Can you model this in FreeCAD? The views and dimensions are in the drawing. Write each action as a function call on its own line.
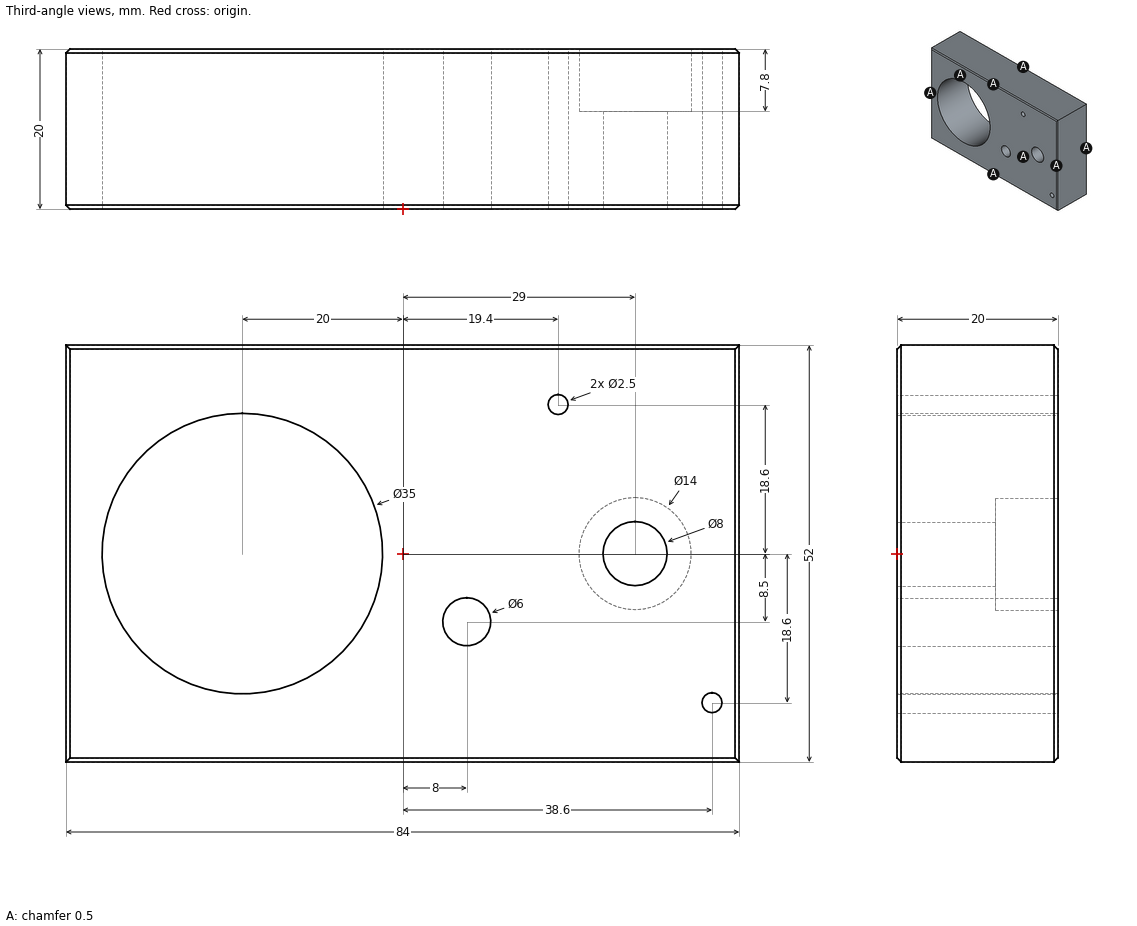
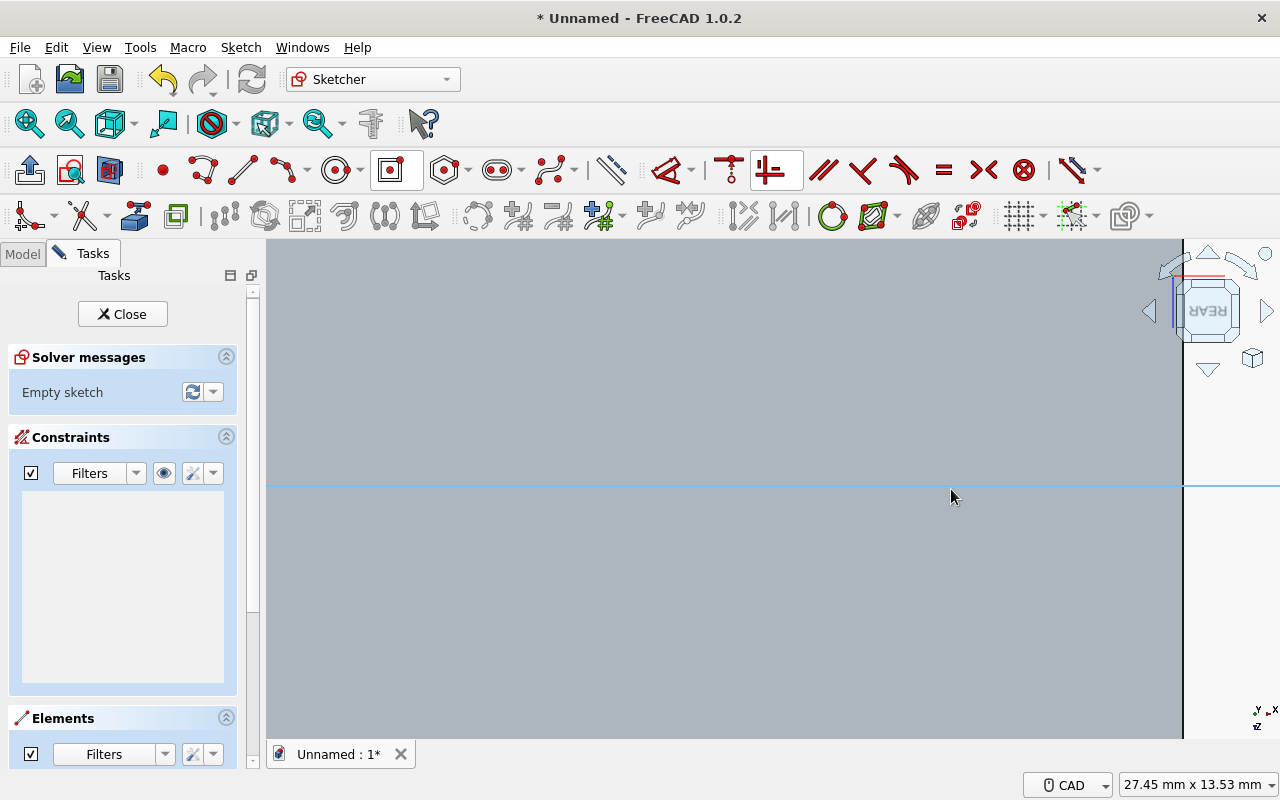
click(336, 170)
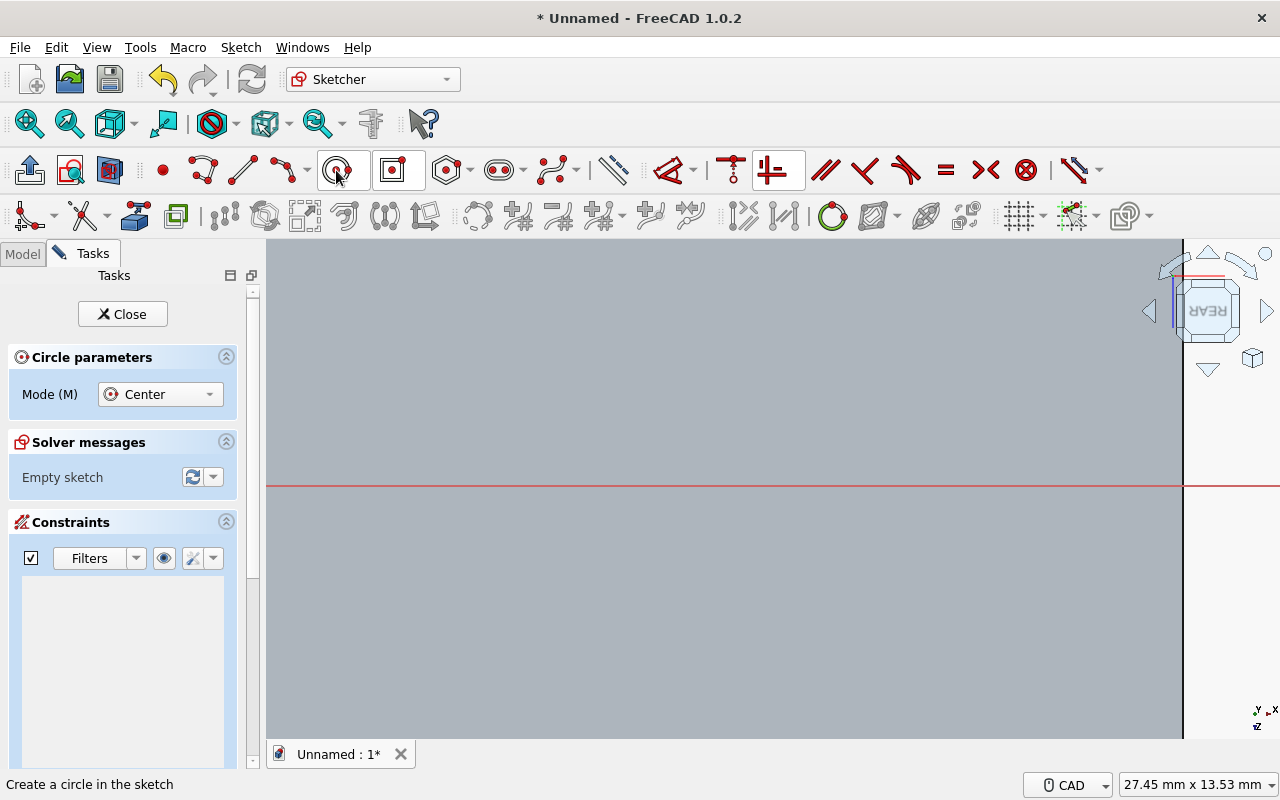
click(703, 486)
move(807, 381)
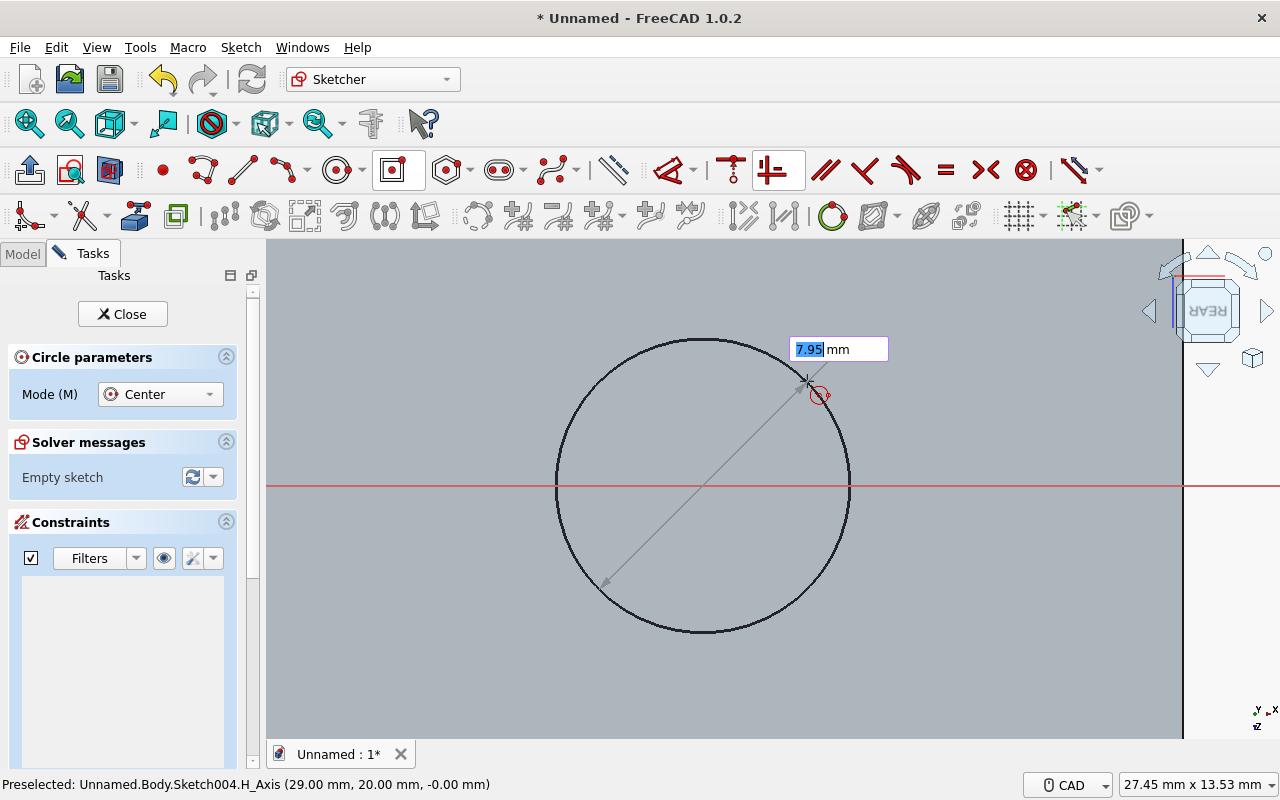
text(8)
key(Return)
key(Escape)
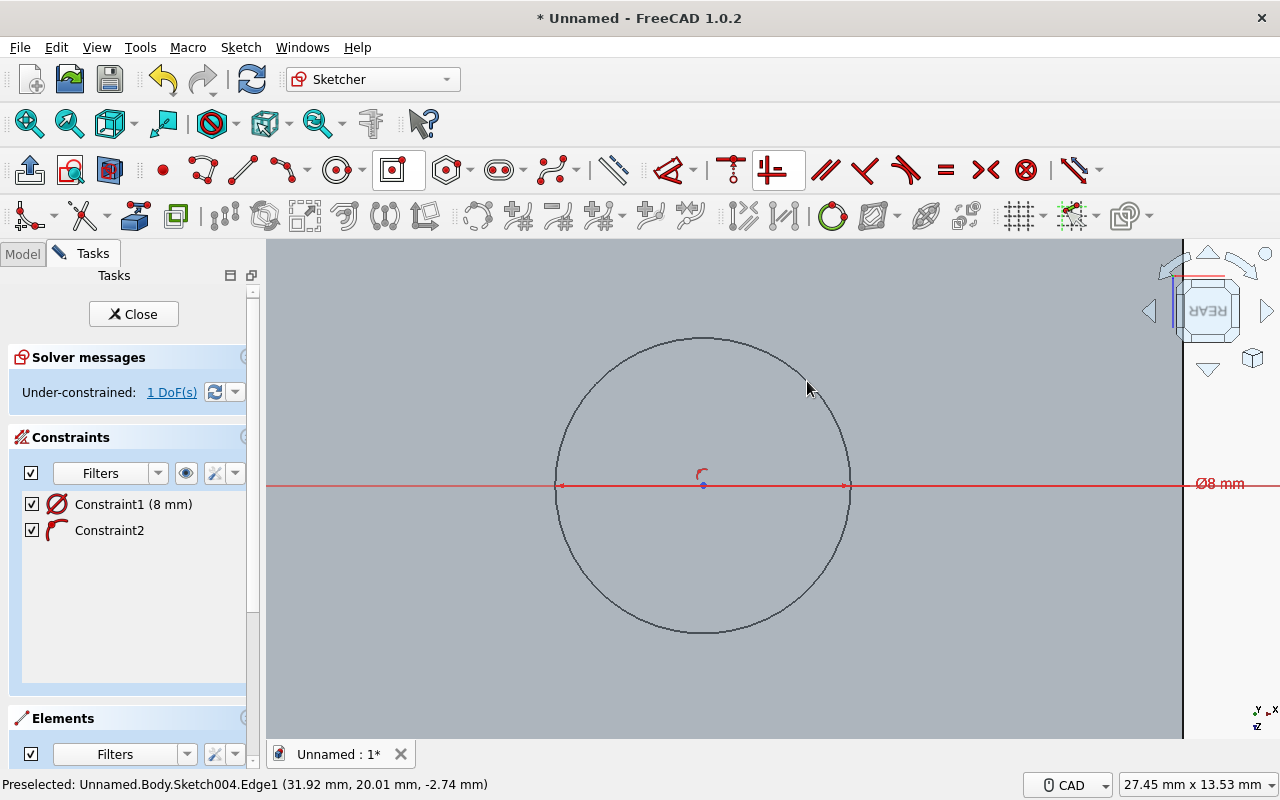
click(668, 170)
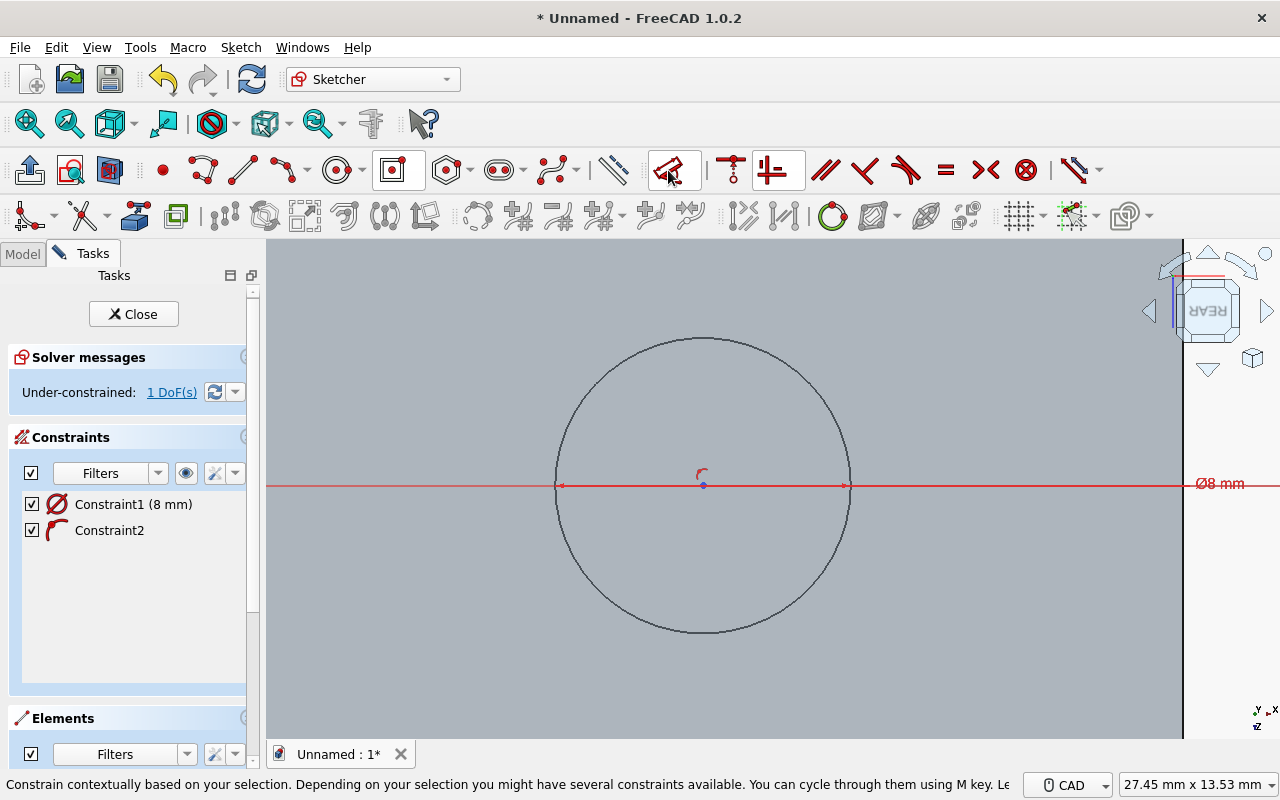
click(703, 486)
click(498, 520)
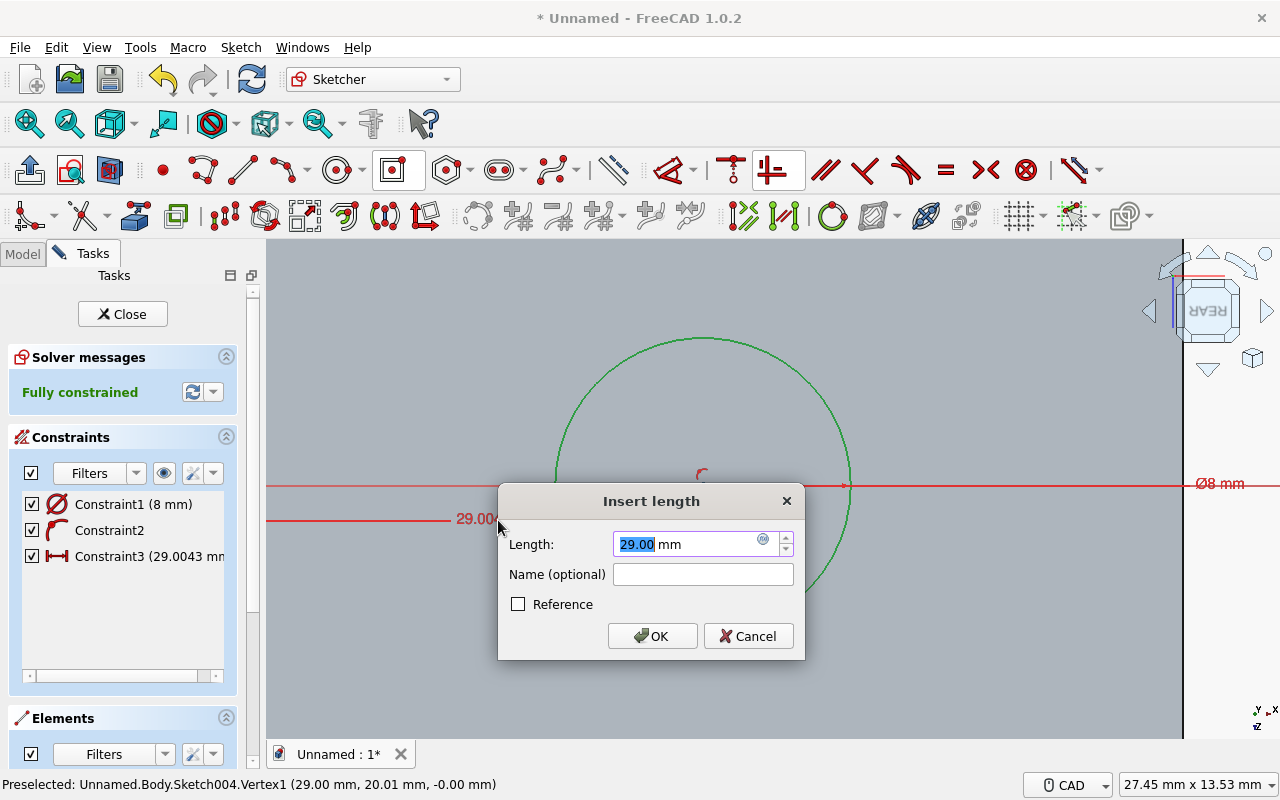
text(29)
key(Return)
key(Escape)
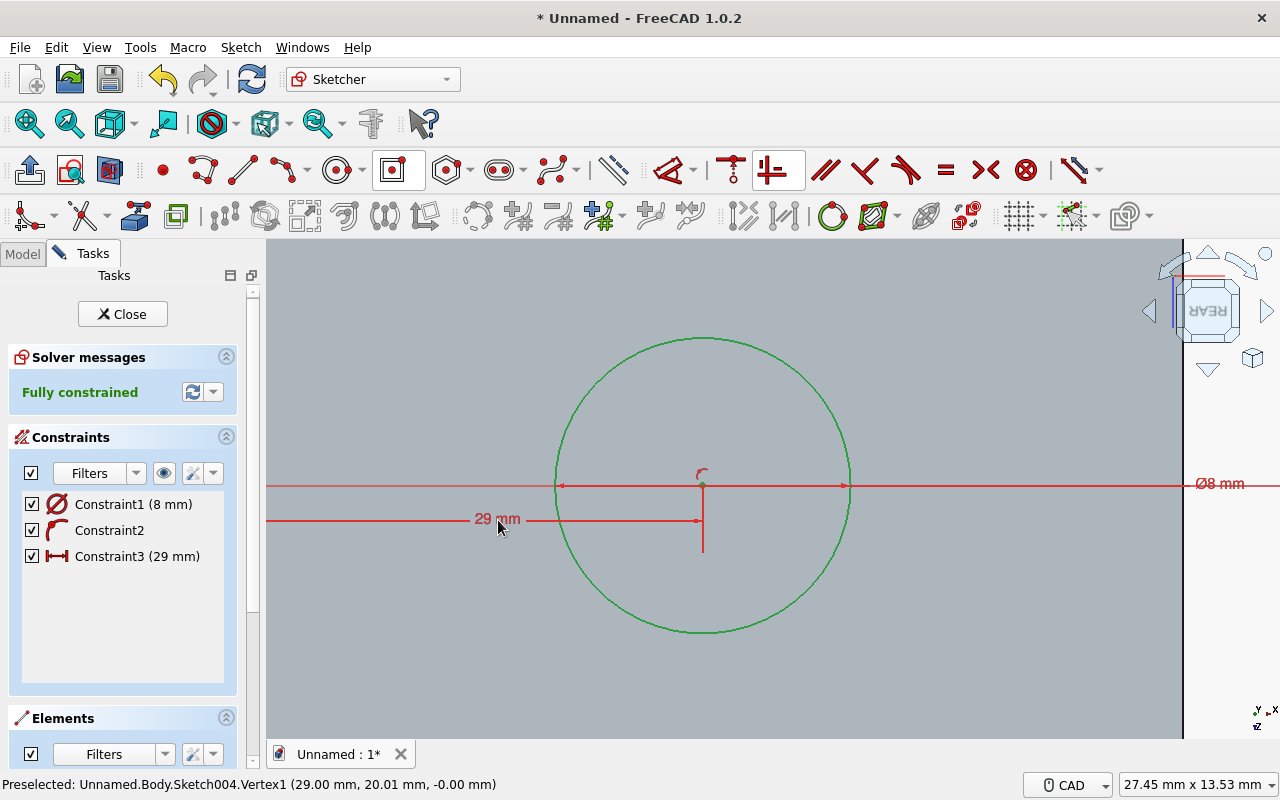
click(123, 314)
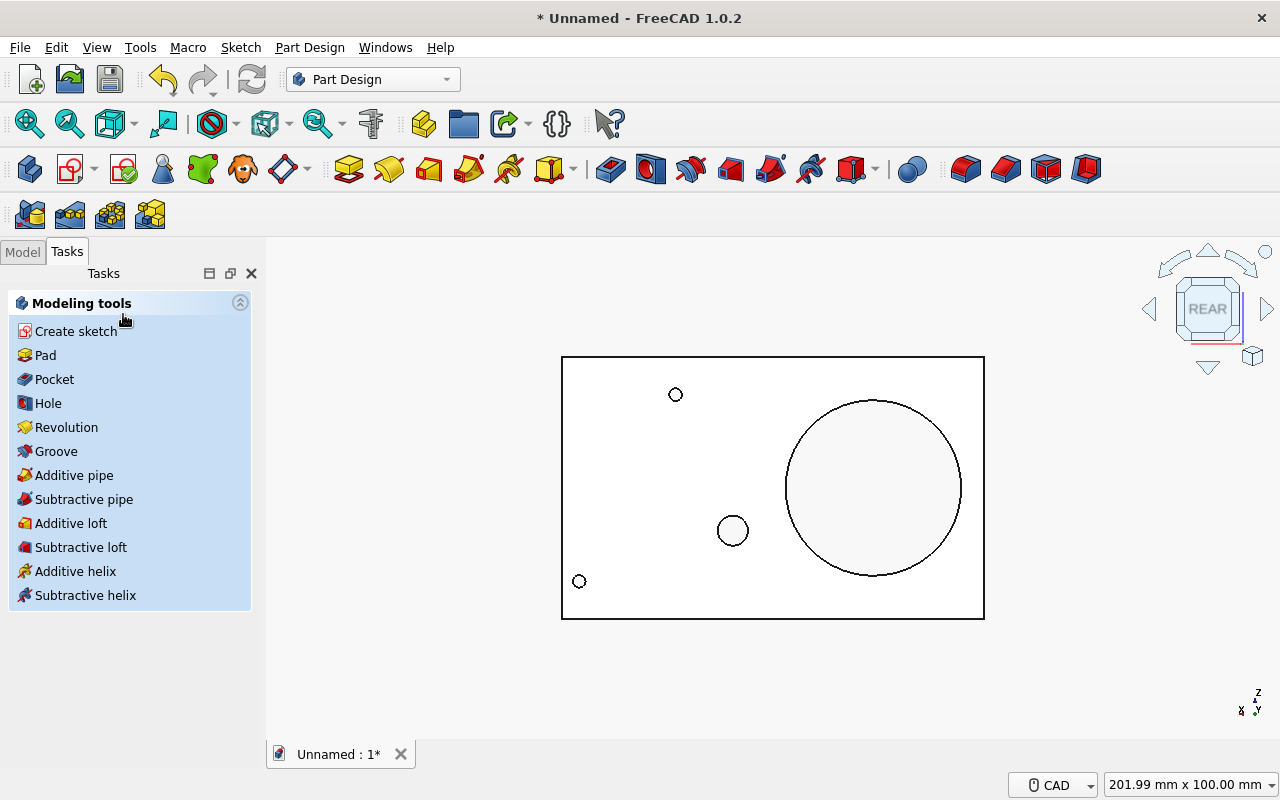
click(612, 170)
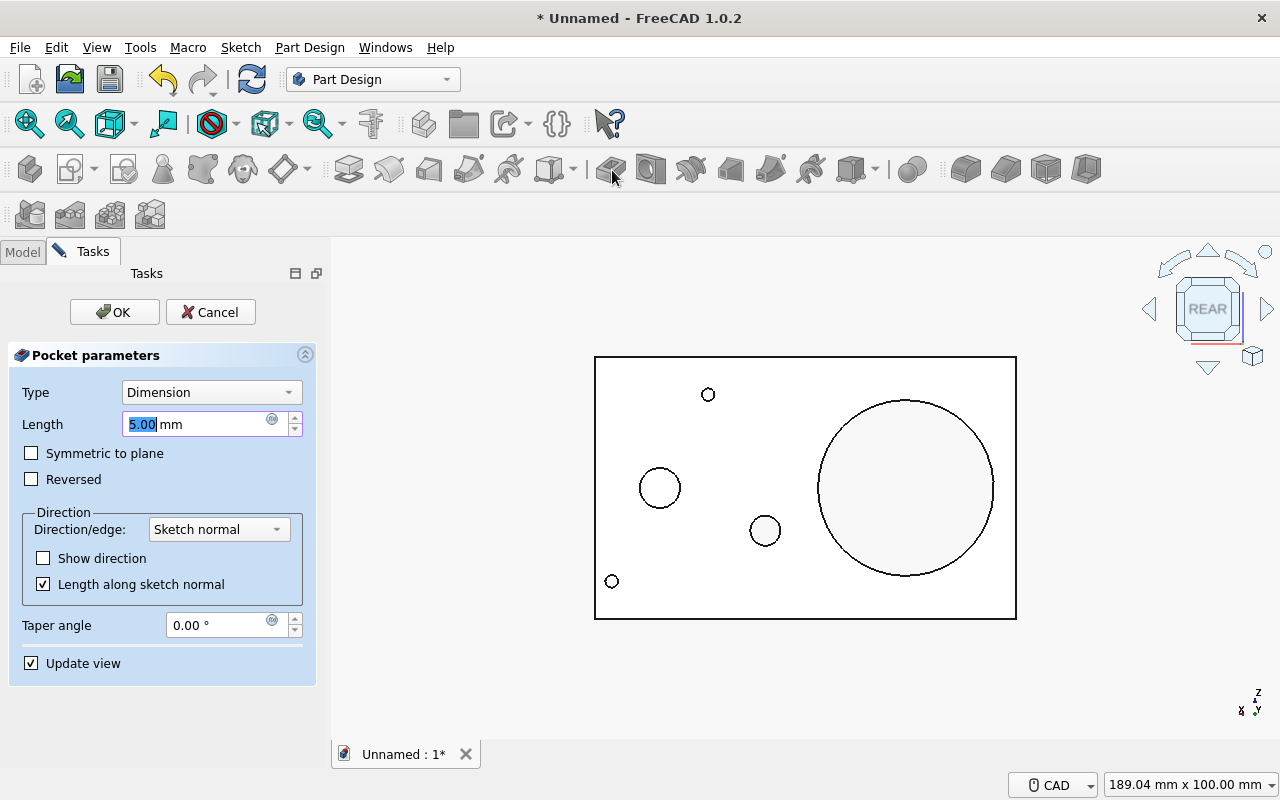
text(20)
key(Tab)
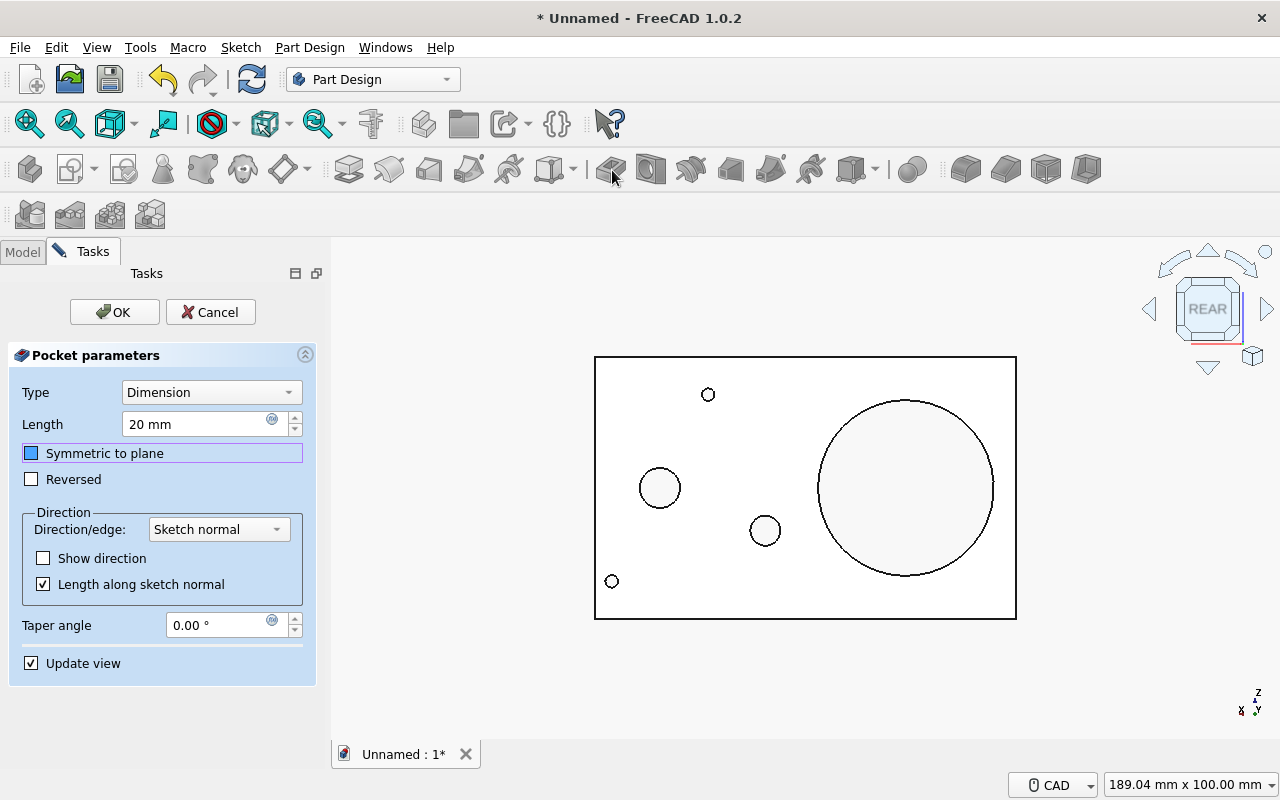
click(115, 312)